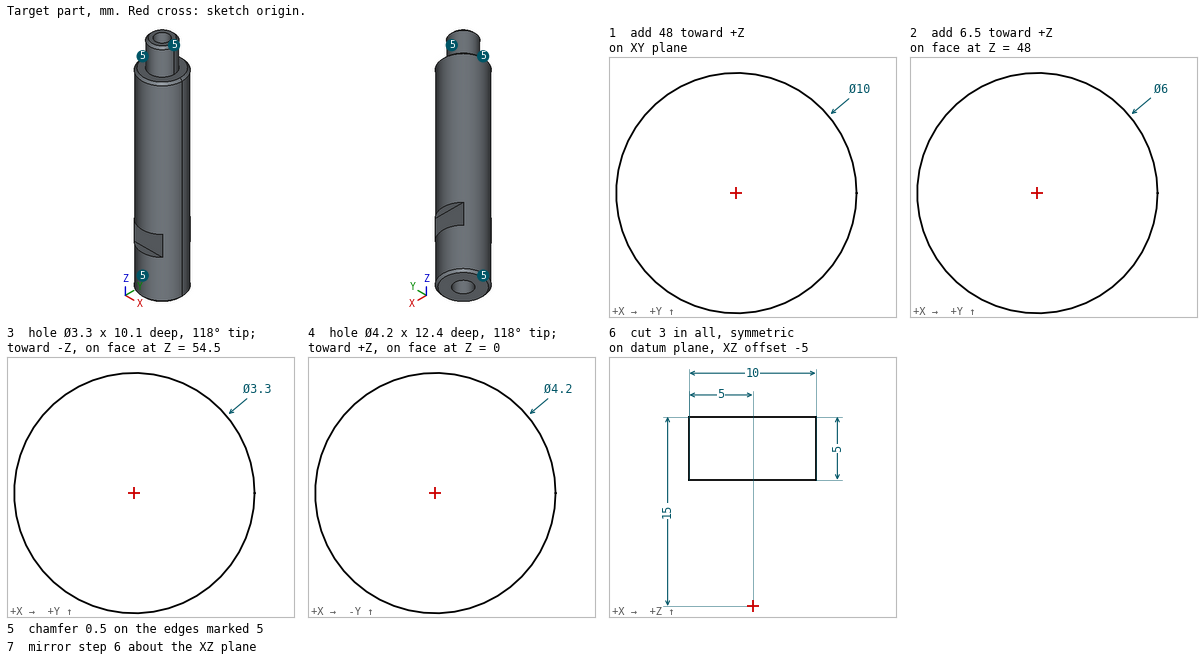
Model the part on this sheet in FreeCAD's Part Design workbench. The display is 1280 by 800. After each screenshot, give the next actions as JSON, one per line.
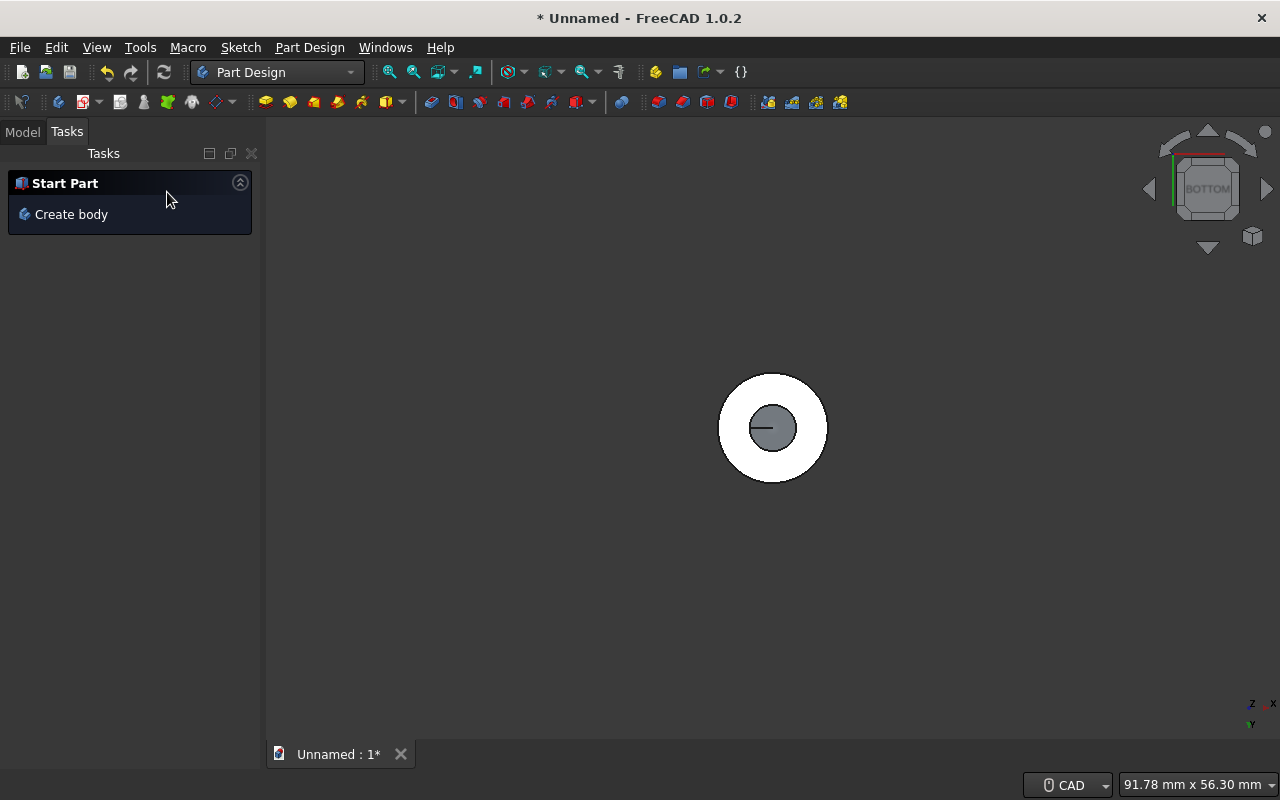
{"action": "left_click", "coordinate": [390, 72]}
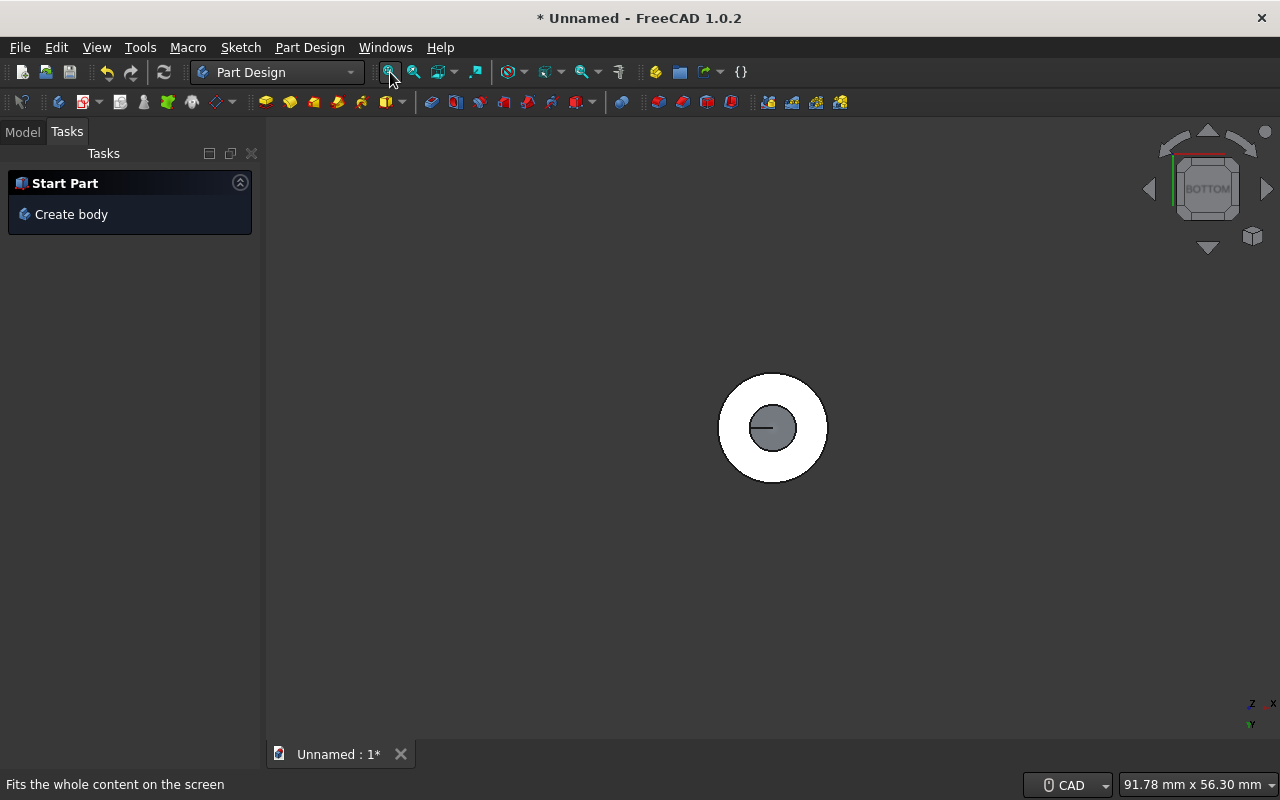
{"action": "left_click", "coordinate": [728, 459]}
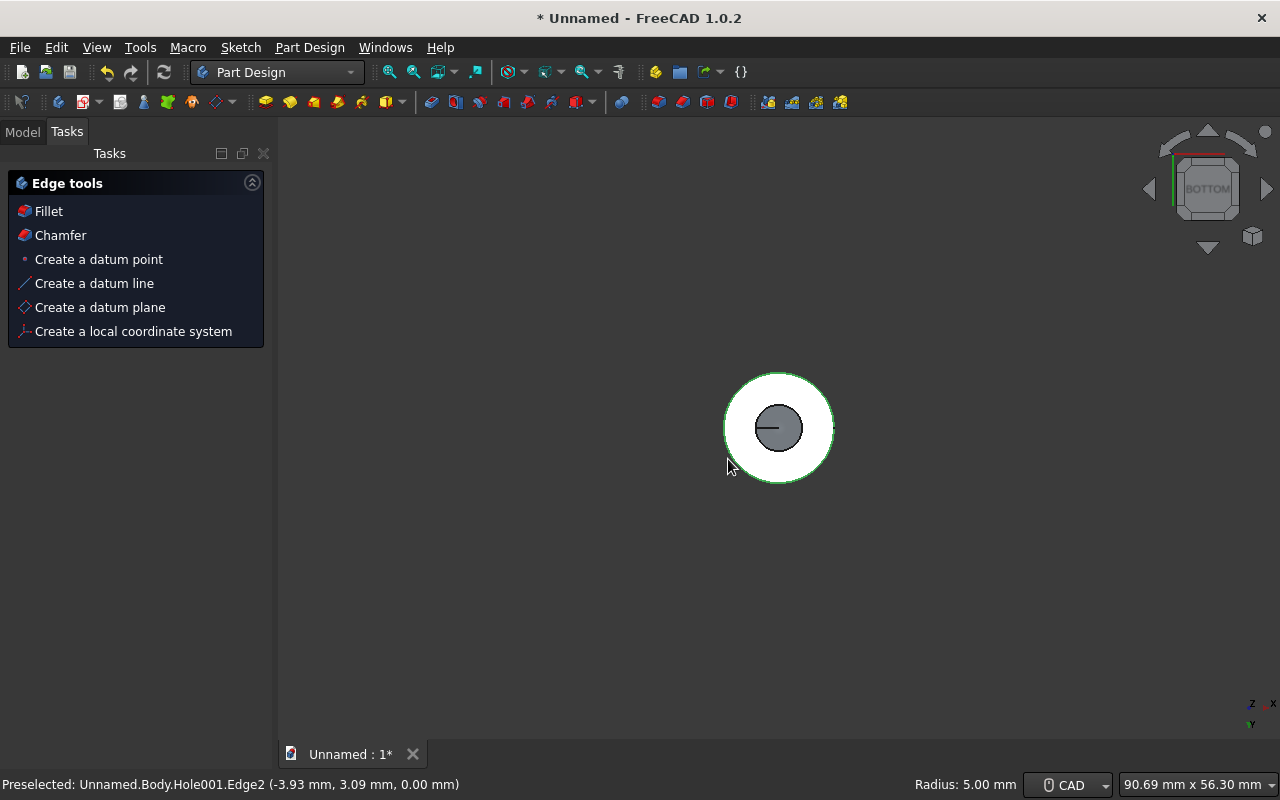
{"action": "key", "text": "0"}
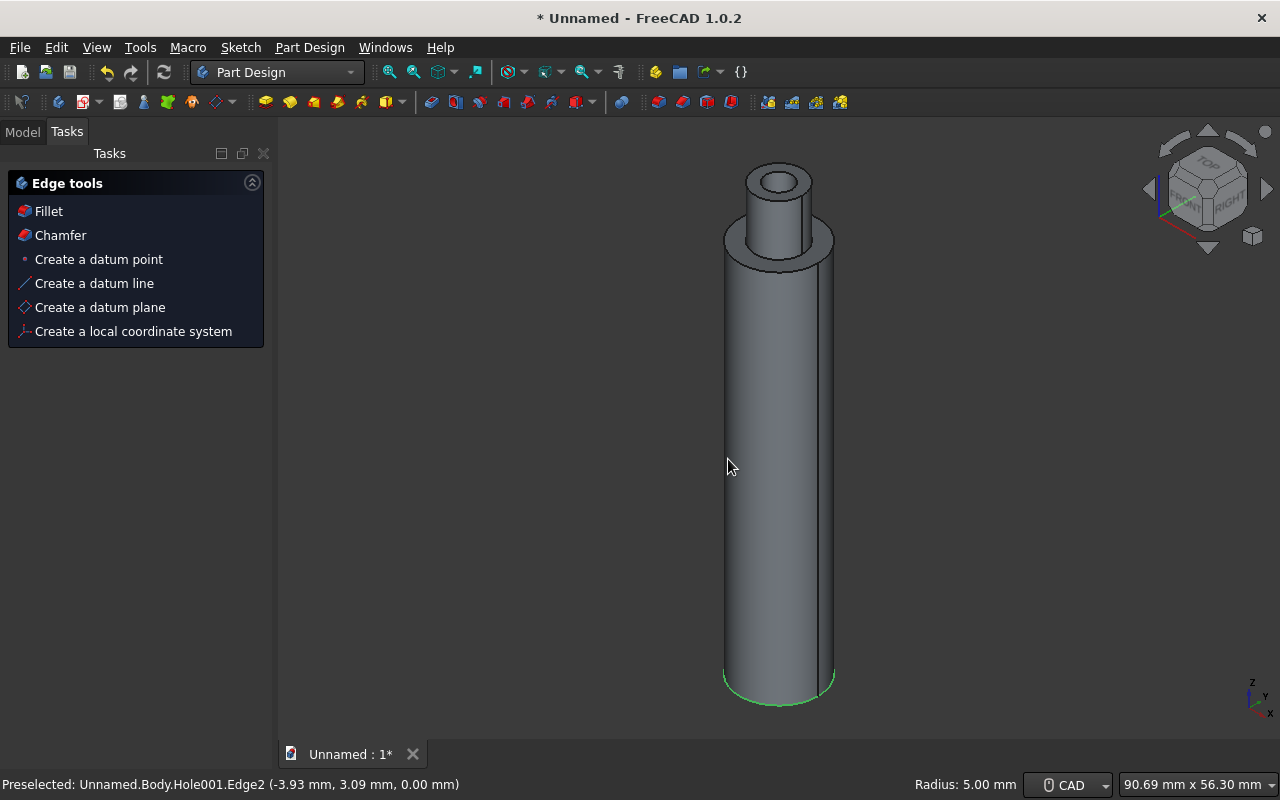
{"action": "left_click", "coordinate": [730, 254], "text": "ctrl"}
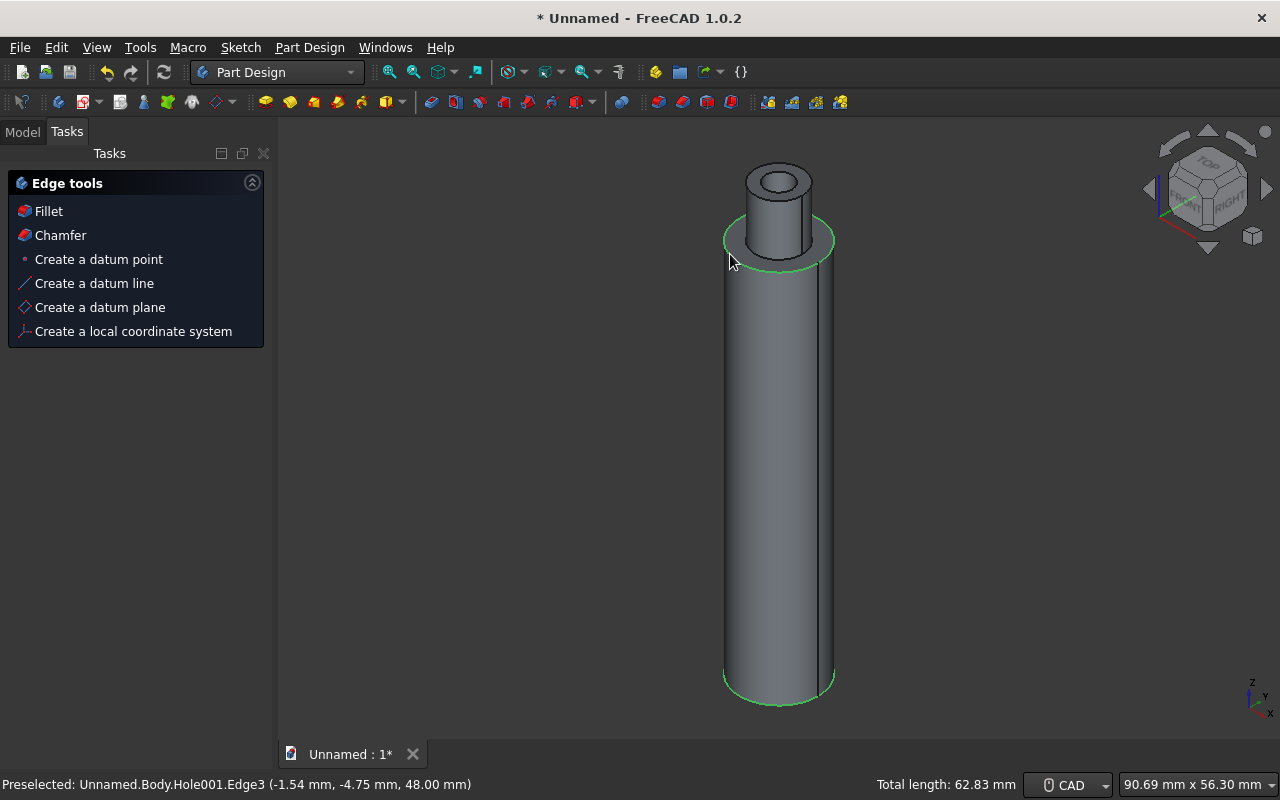
{"action": "left_click", "coordinate": [749, 190], "text": "ctrl"}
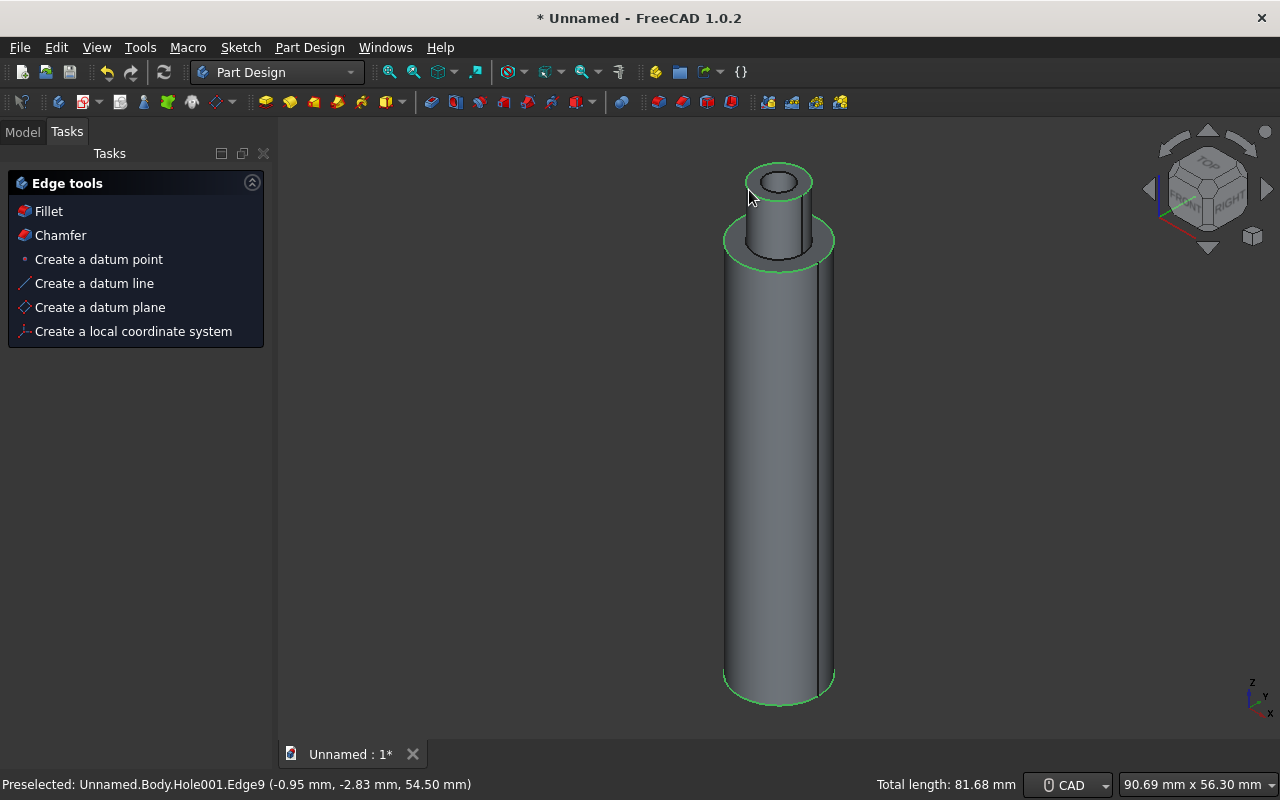
{"action": "left_click", "coordinate": [684, 102]}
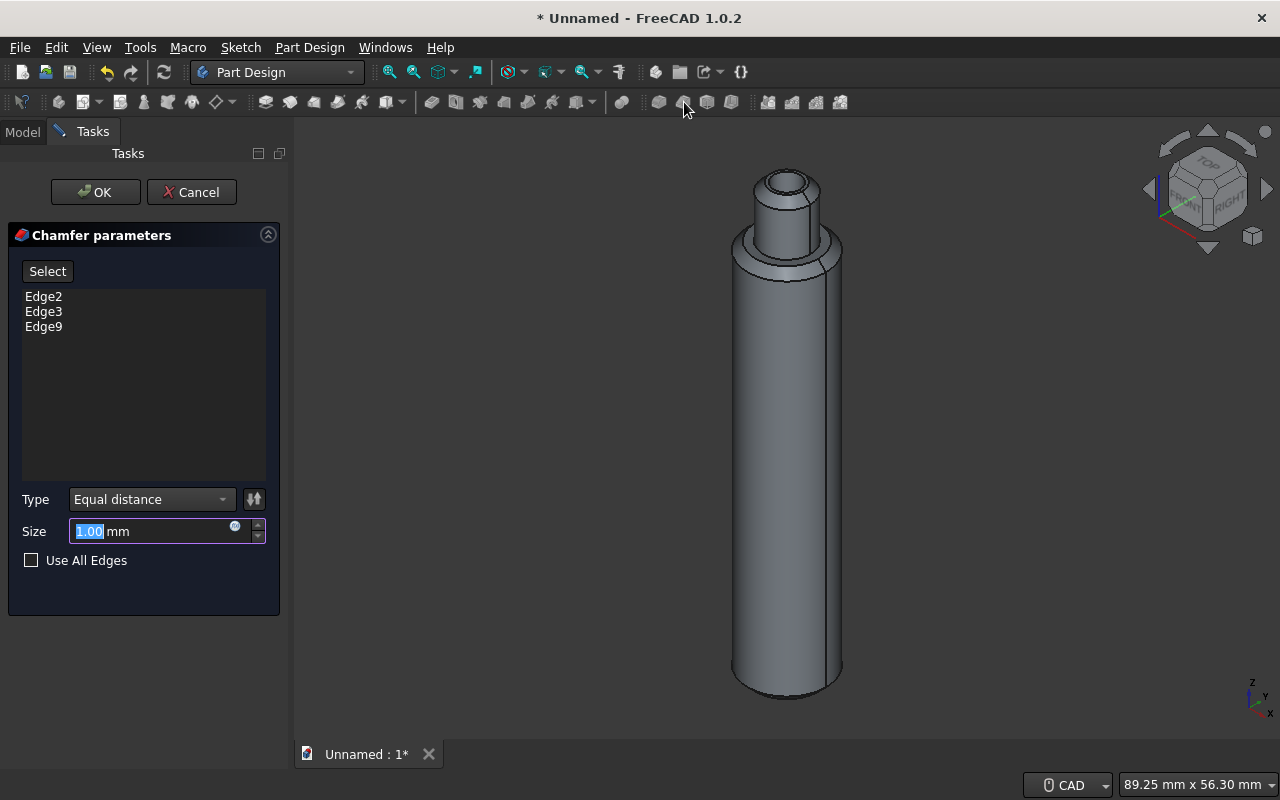
{"action": "type", "text": "0.5"}
{"action": "key", "text": "Tab"}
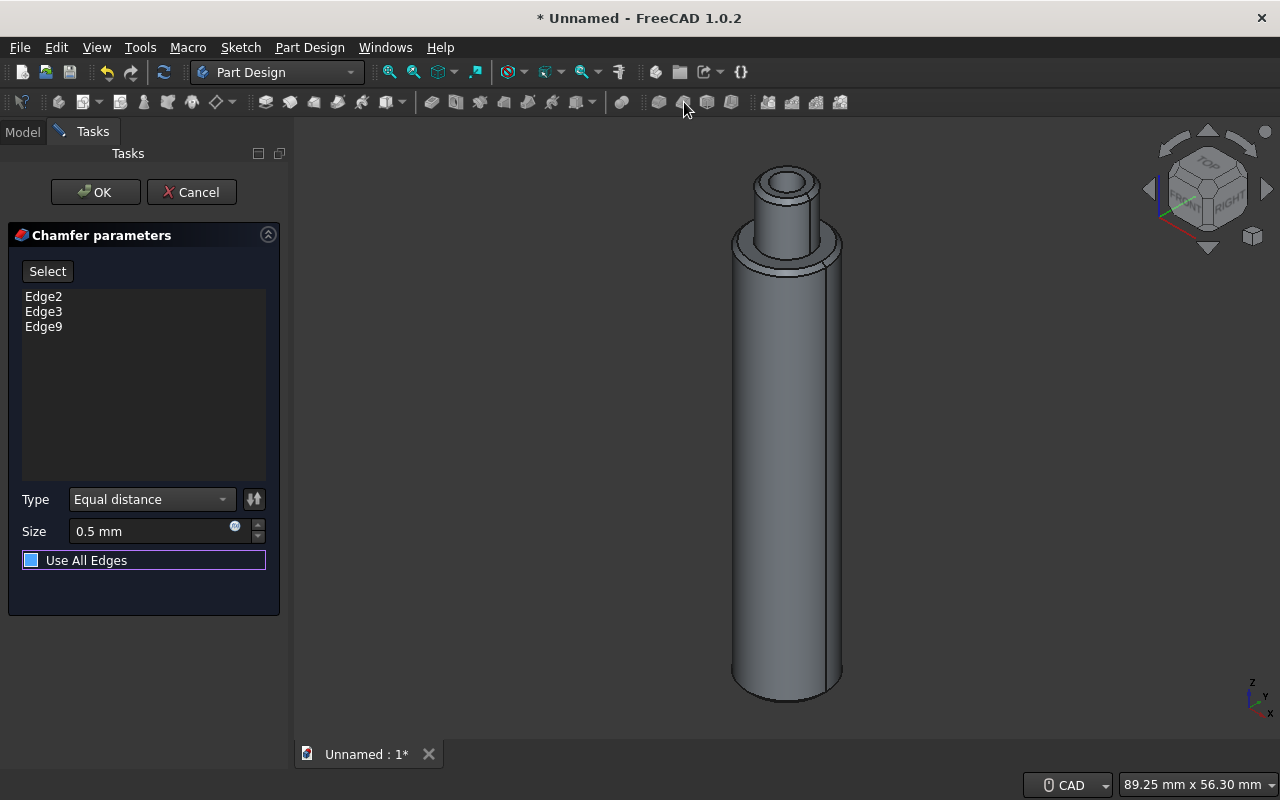
{"action": "left_click", "coordinate": [96, 192]}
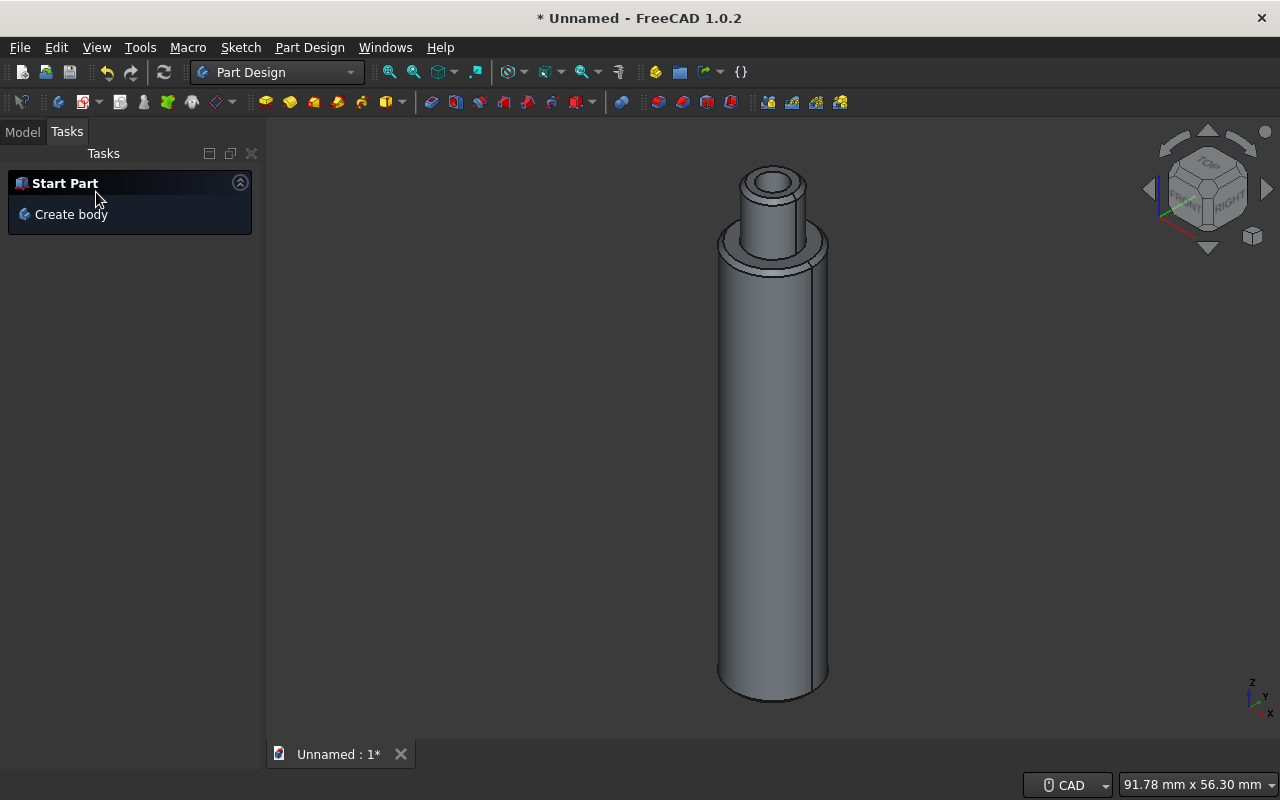
{"action": "left_click", "coordinate": [23, 131]}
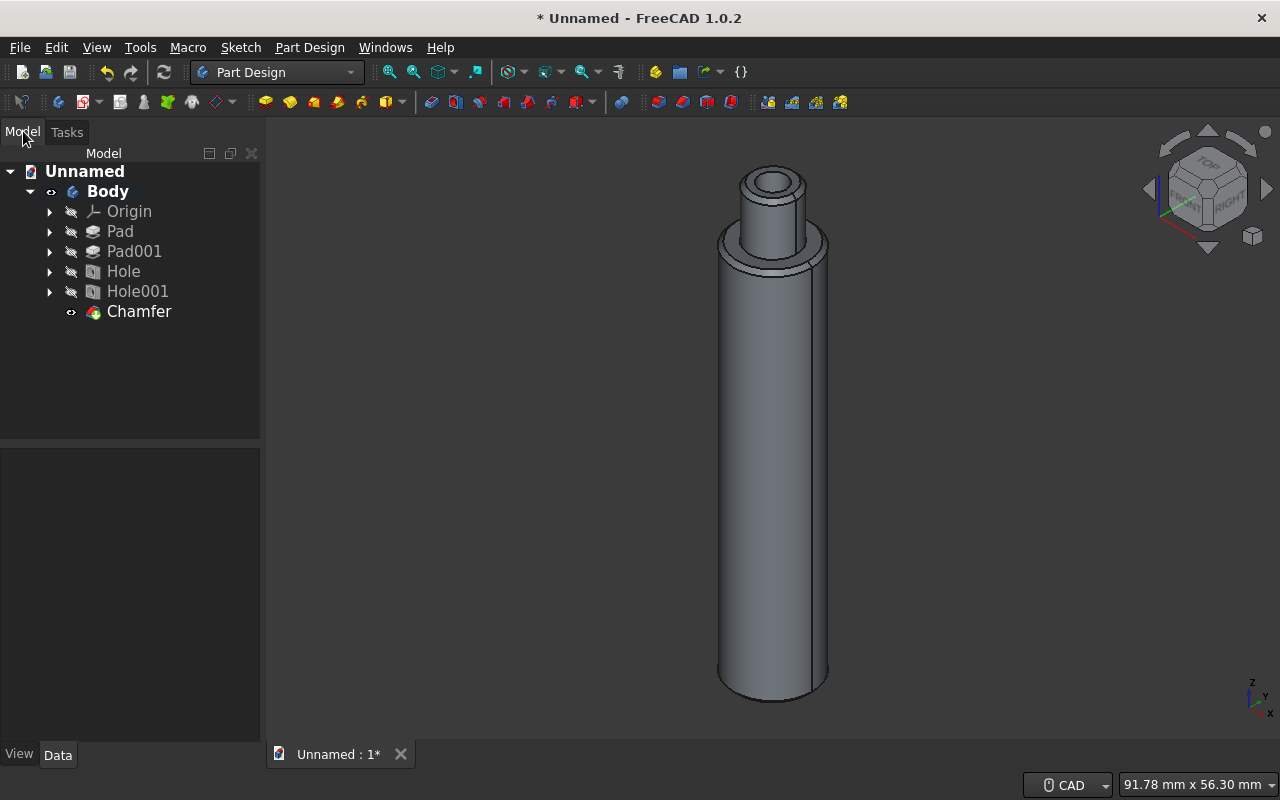
{"action": "left_click", "coordinate": [50, 212]}